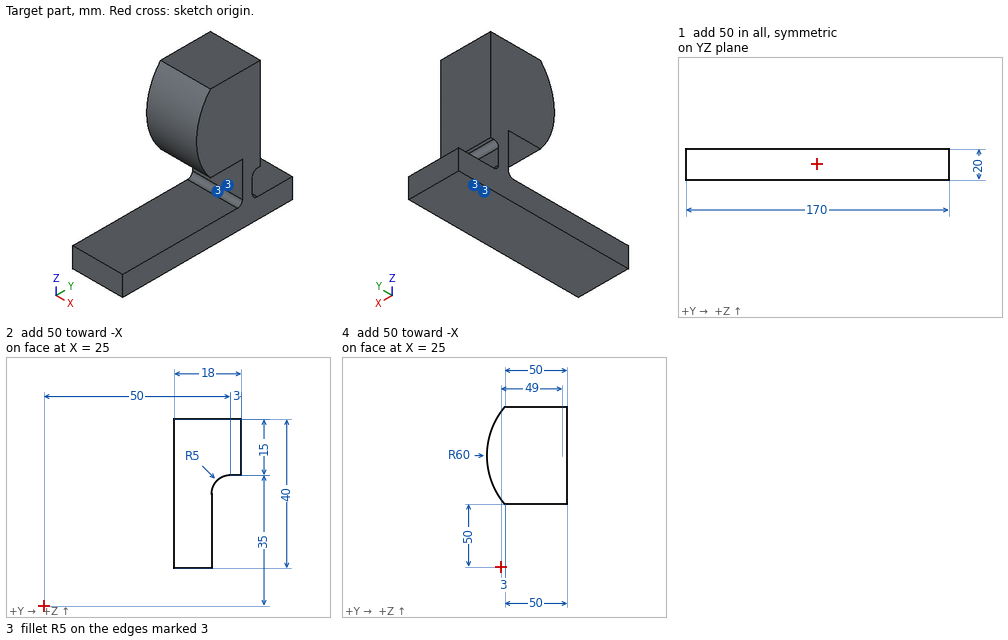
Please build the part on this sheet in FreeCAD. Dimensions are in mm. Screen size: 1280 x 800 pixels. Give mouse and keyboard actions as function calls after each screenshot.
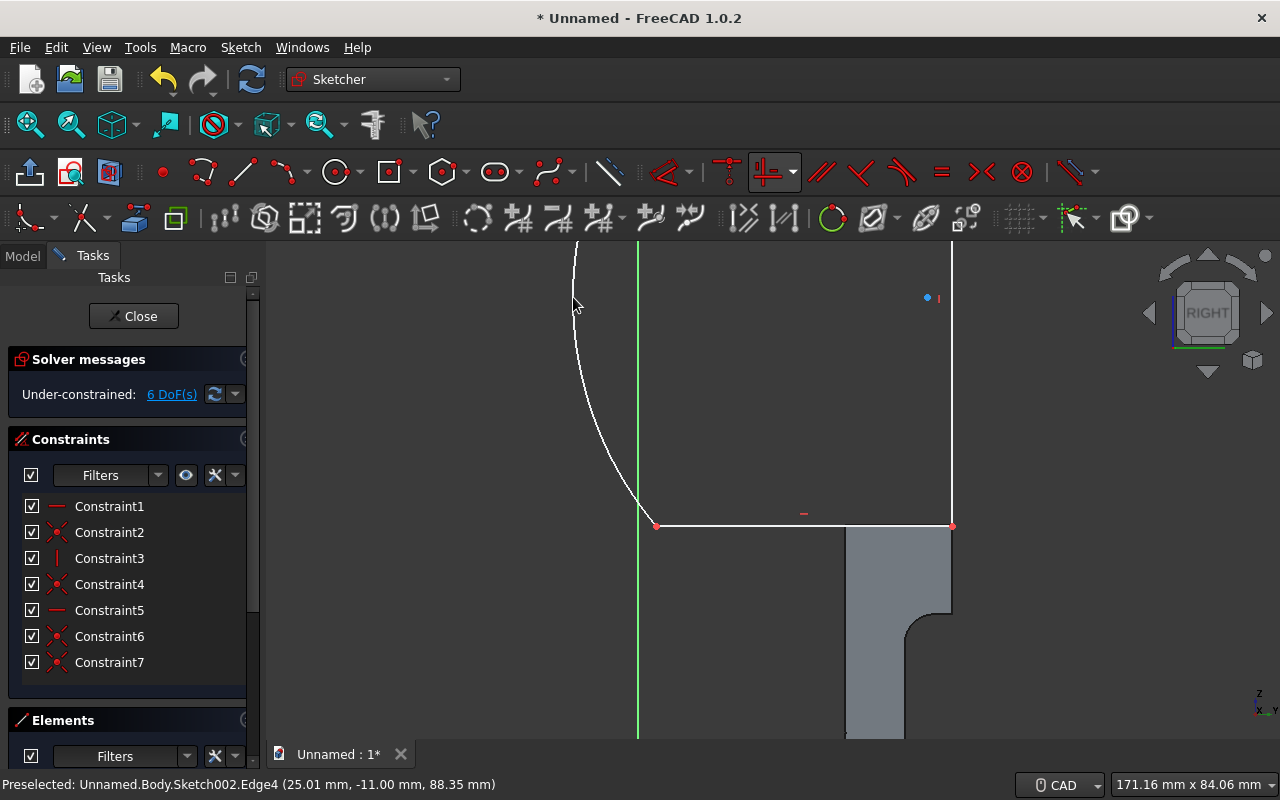
key(d)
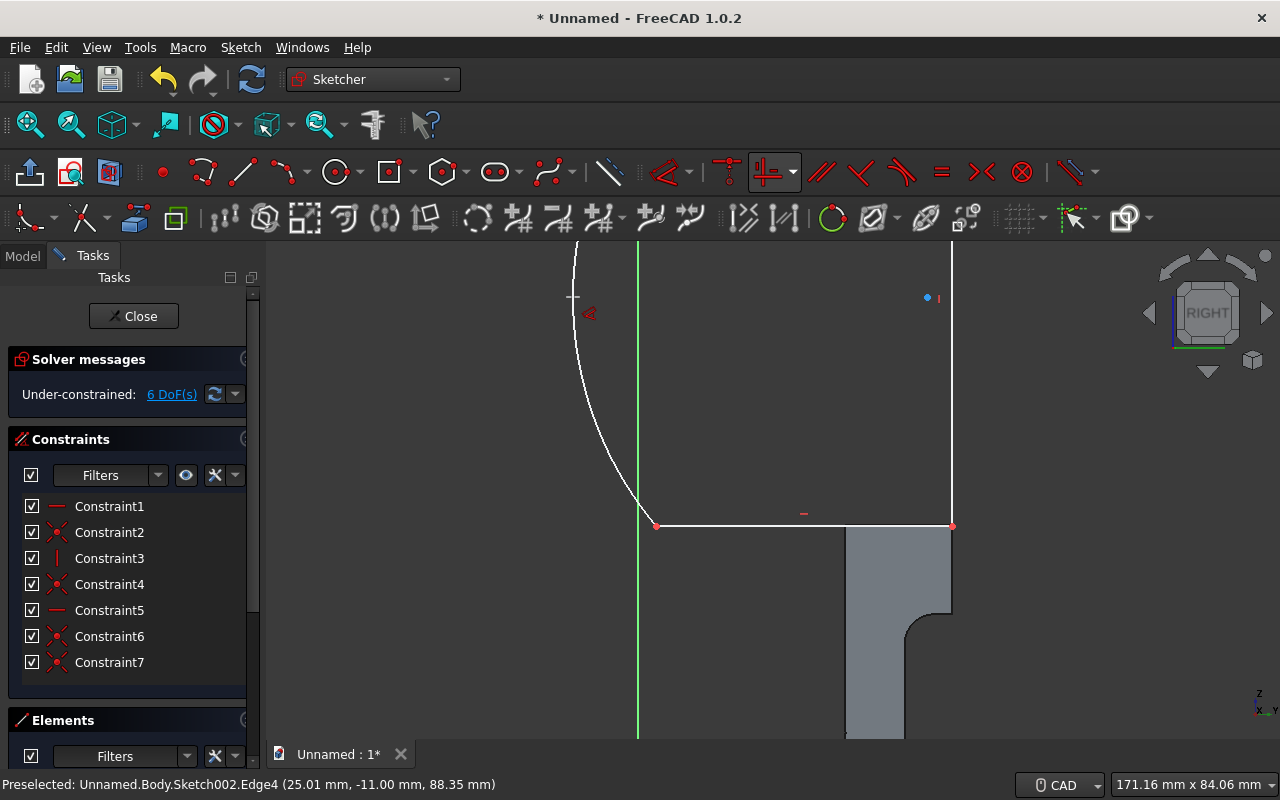
click(587, 396)
click(556, 405)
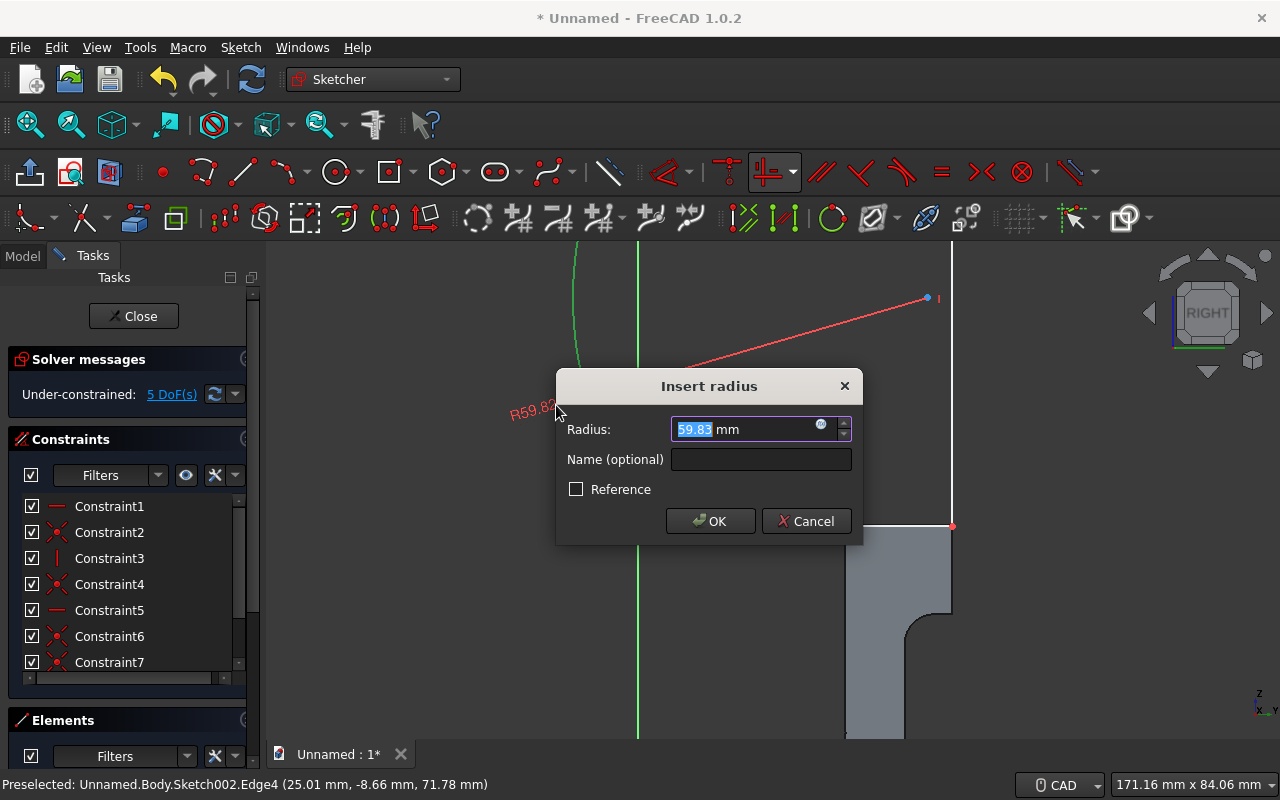
text(60)
key(Return)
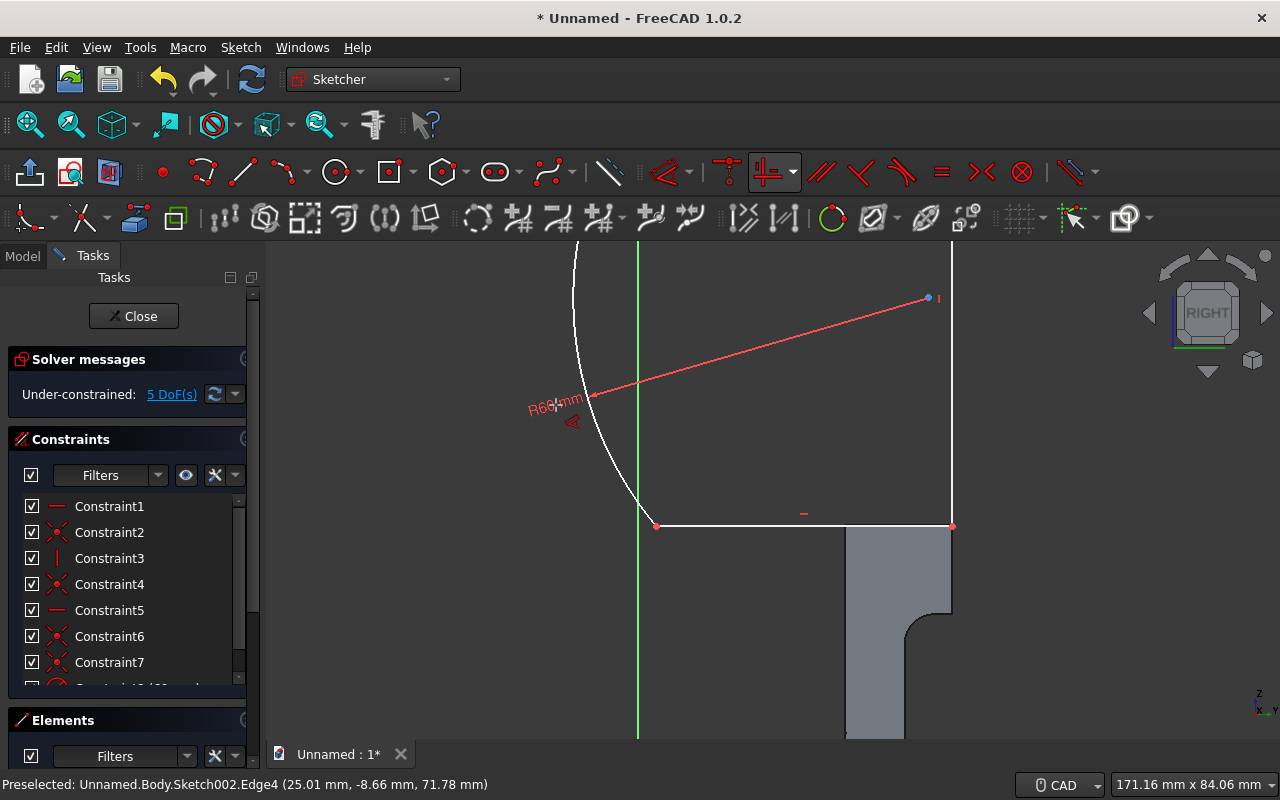
click(745, 526)
click(804, 560)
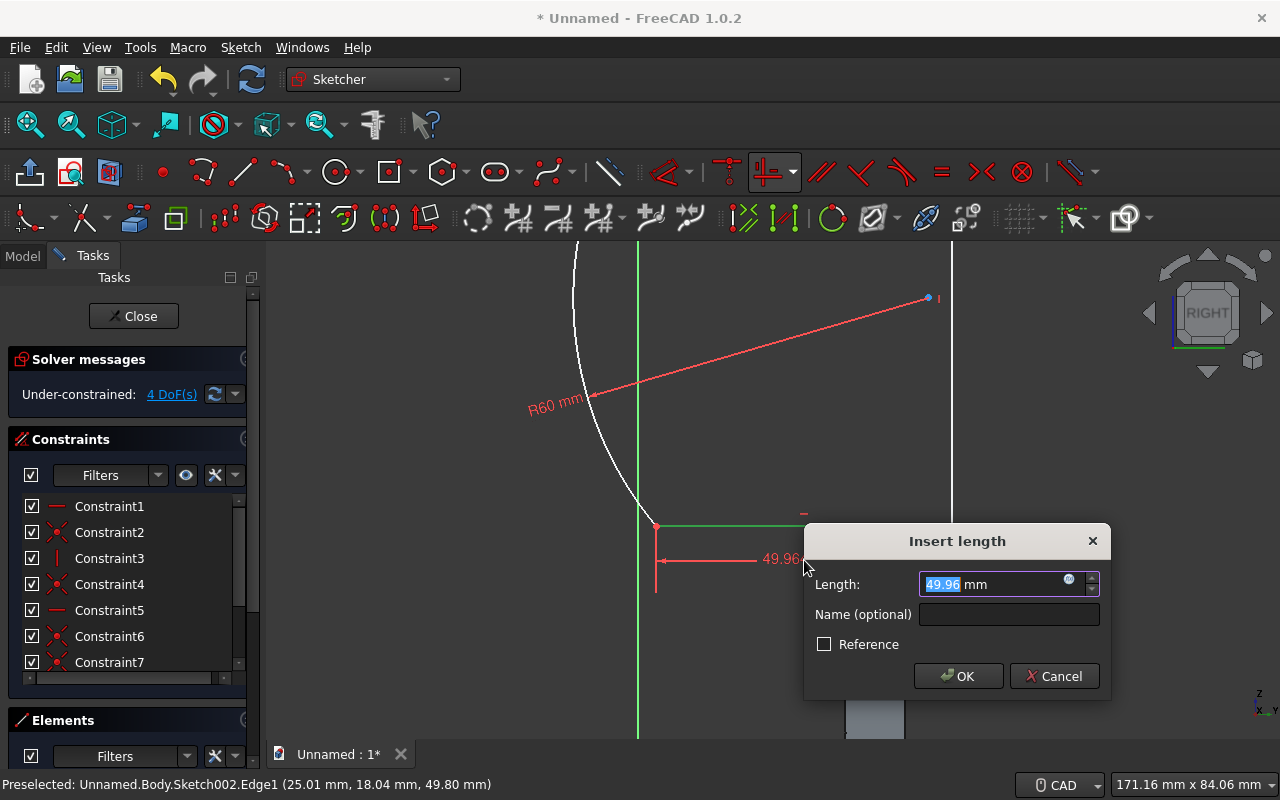
text(50)
key(Return)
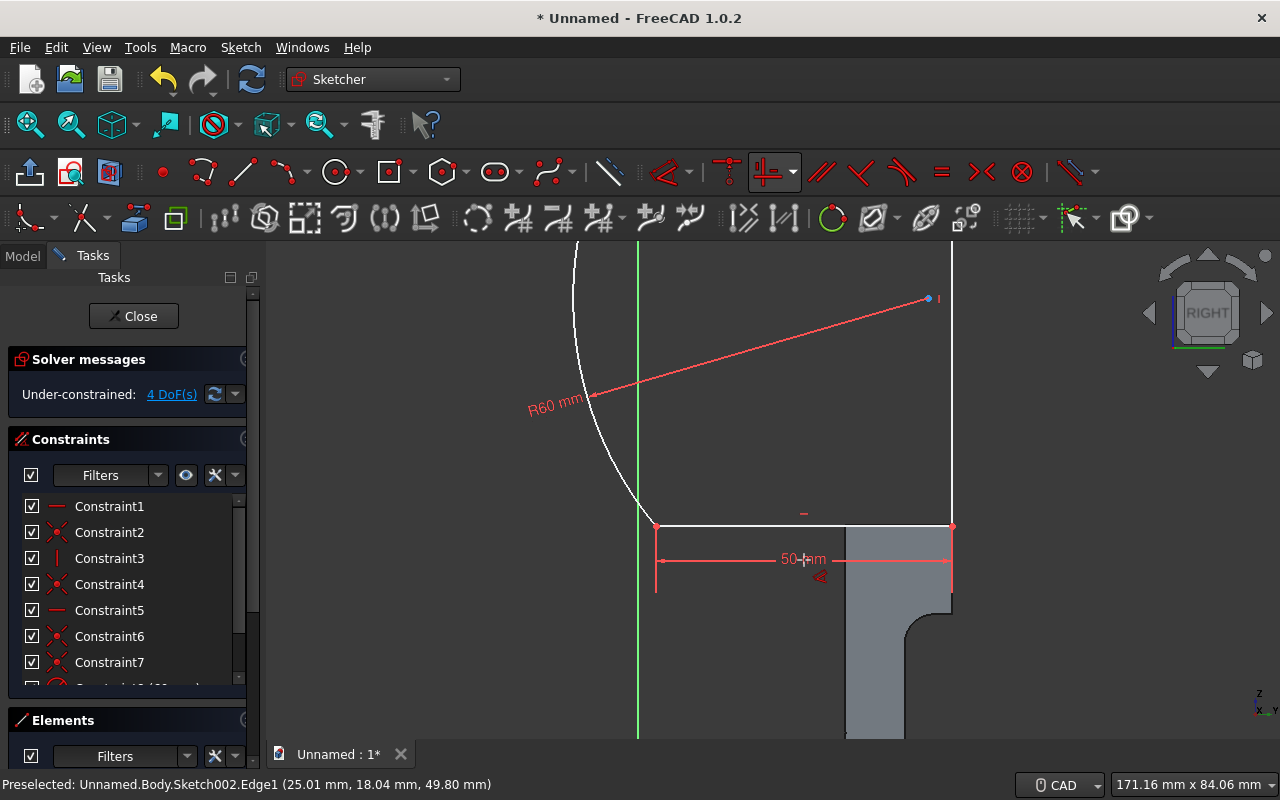
scroll(657, 527, down, 4)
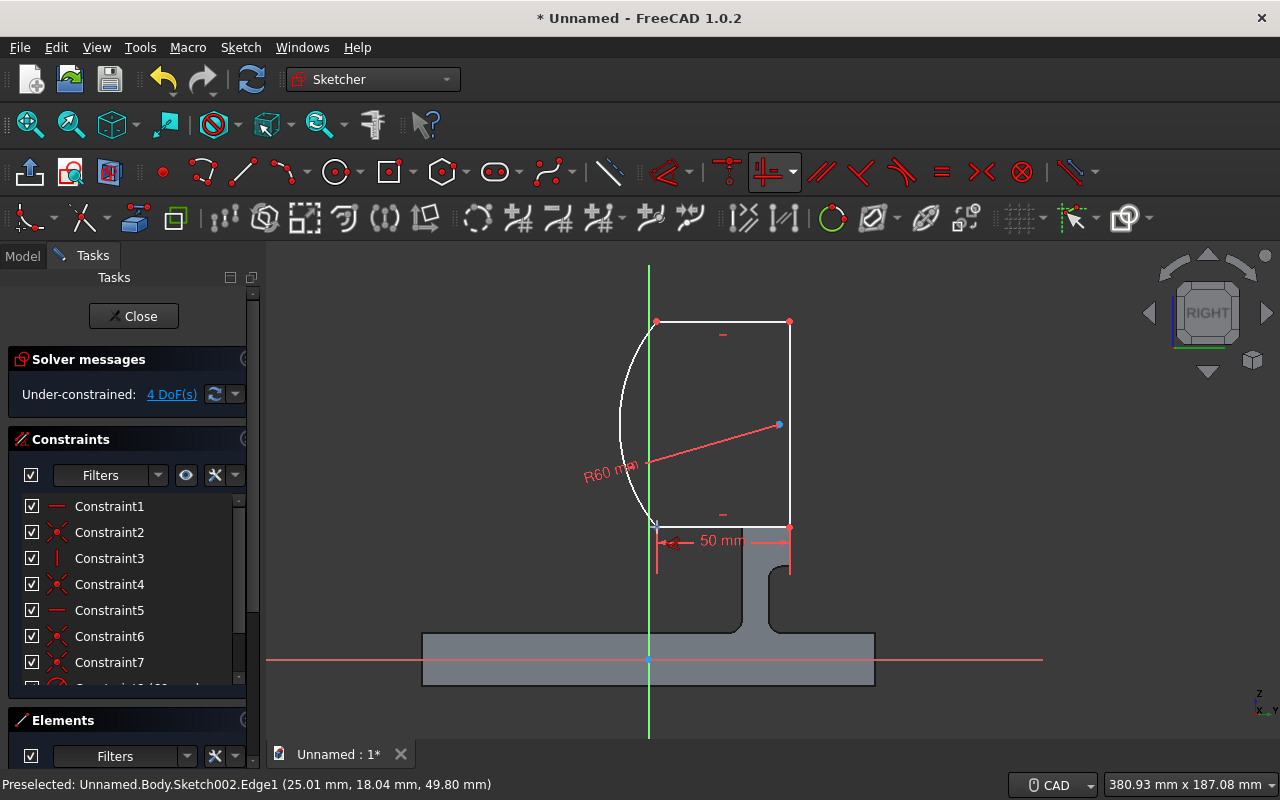
click(750, 322)
click(723, 288)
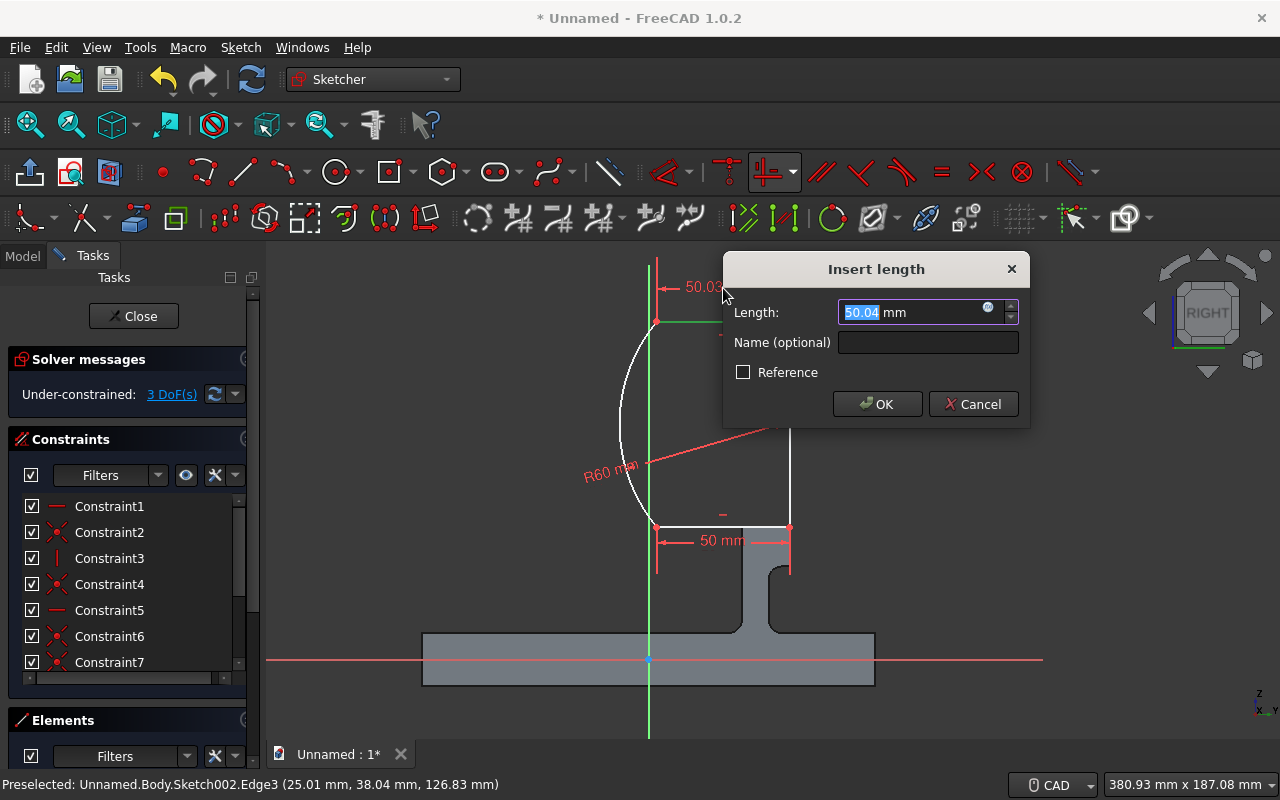
text(50)
key(Return)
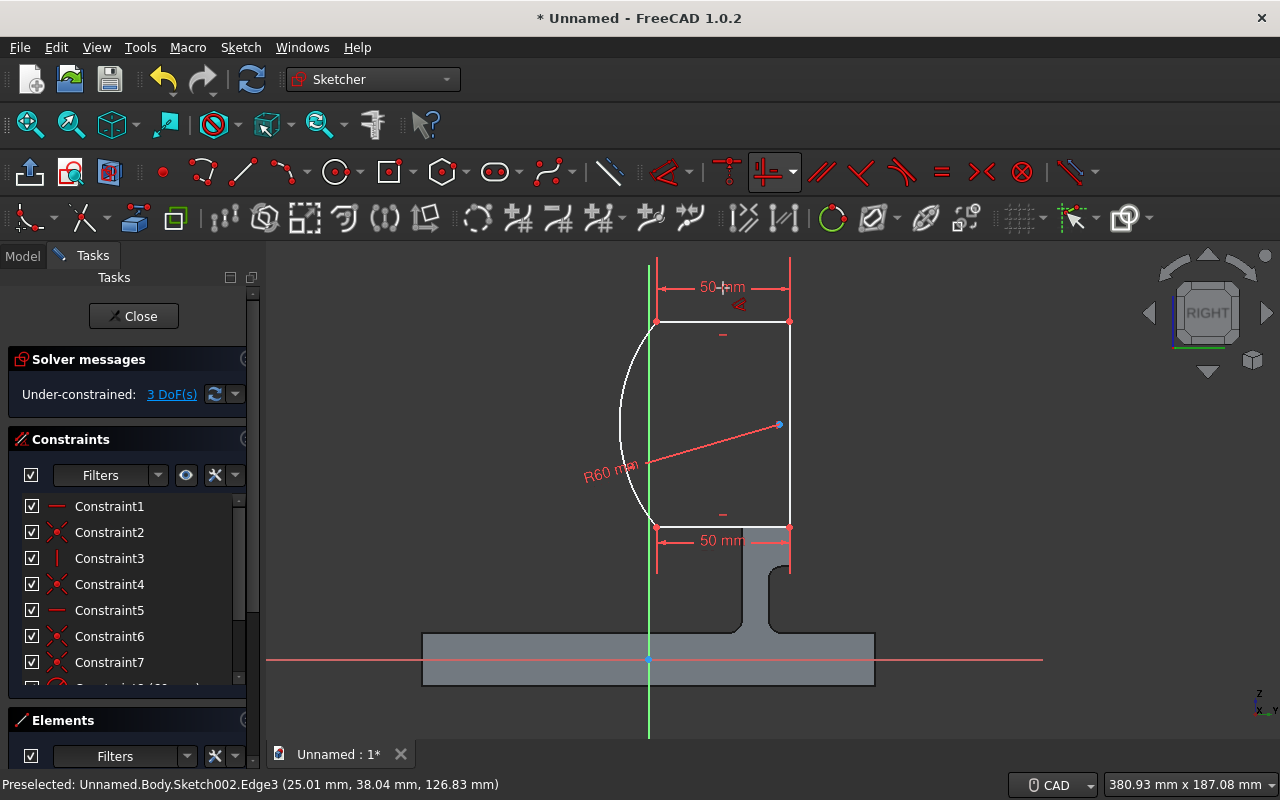
scroll(657, 527, up, 9)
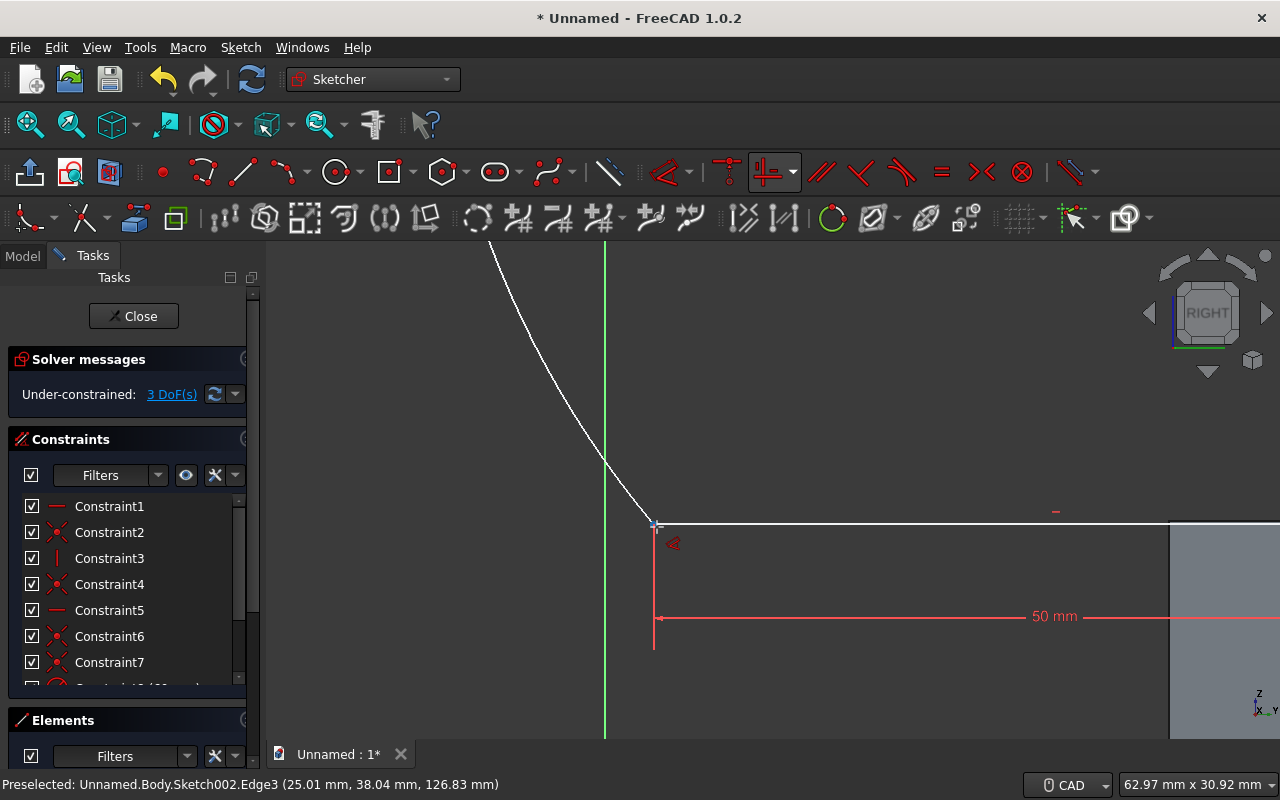
click(654, 524)
click(646, 490)